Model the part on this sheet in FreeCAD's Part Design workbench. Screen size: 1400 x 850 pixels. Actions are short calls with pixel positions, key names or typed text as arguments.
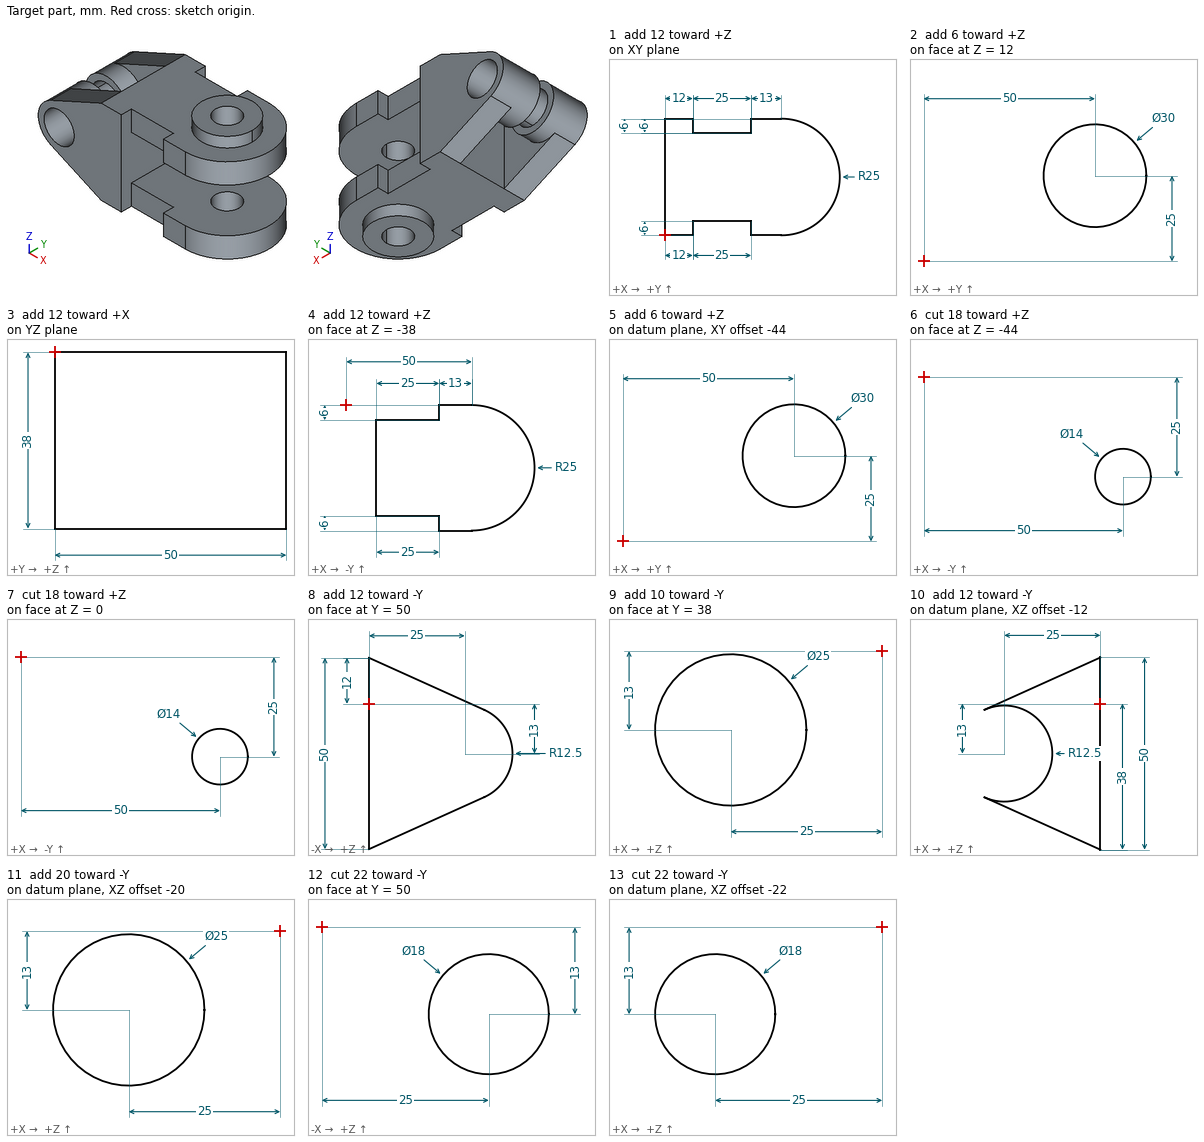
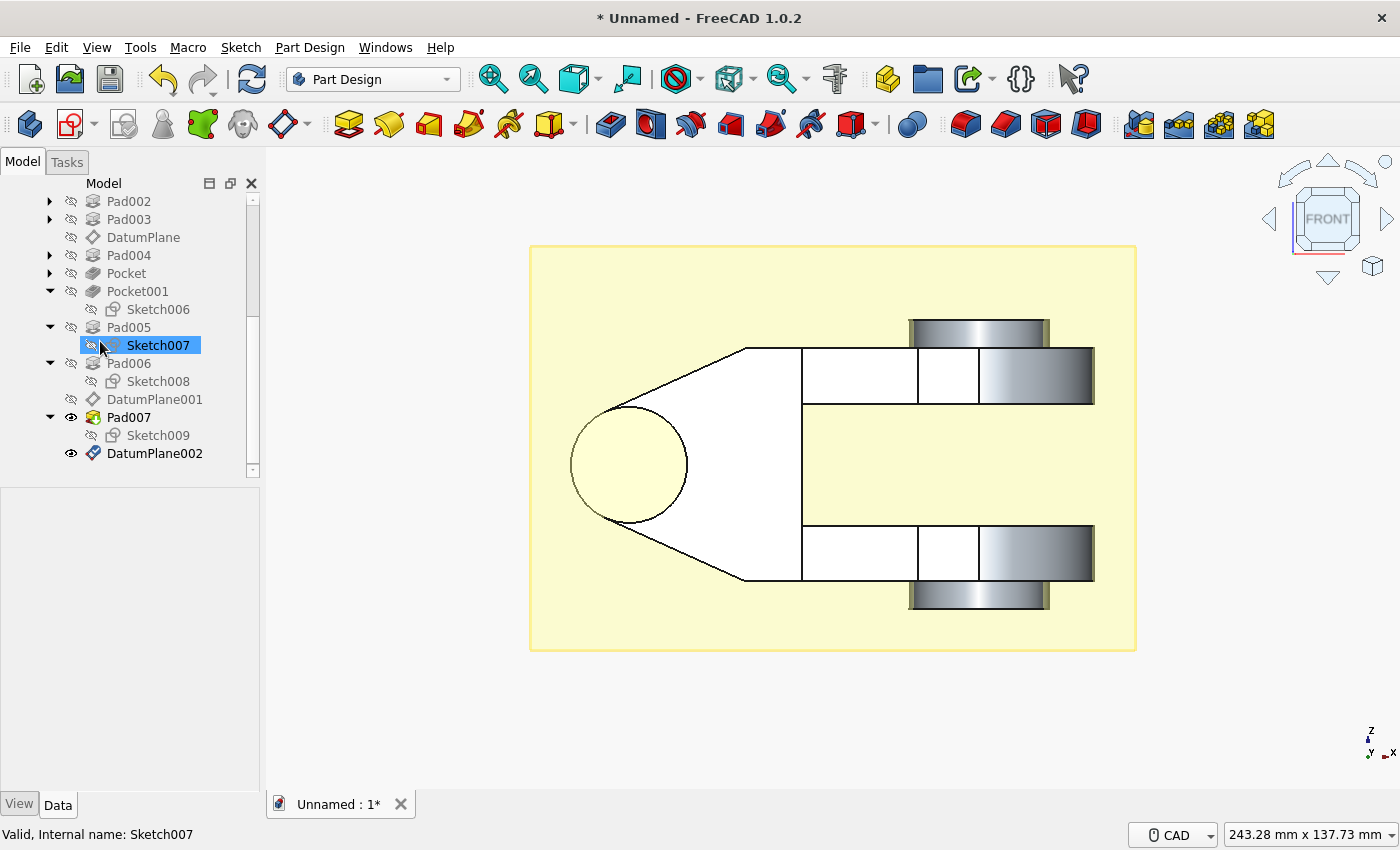
click(116, 453)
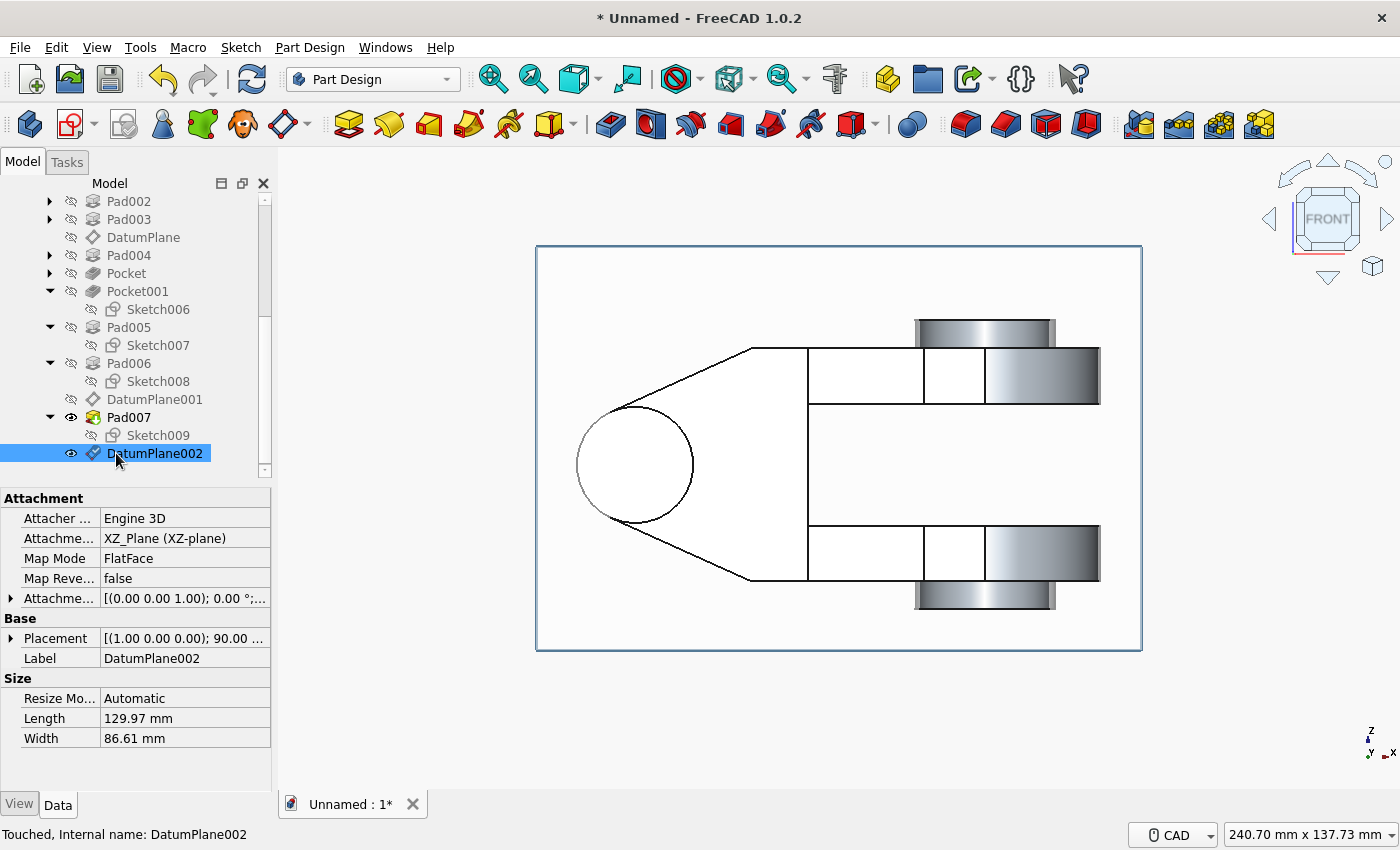
click(70, 124)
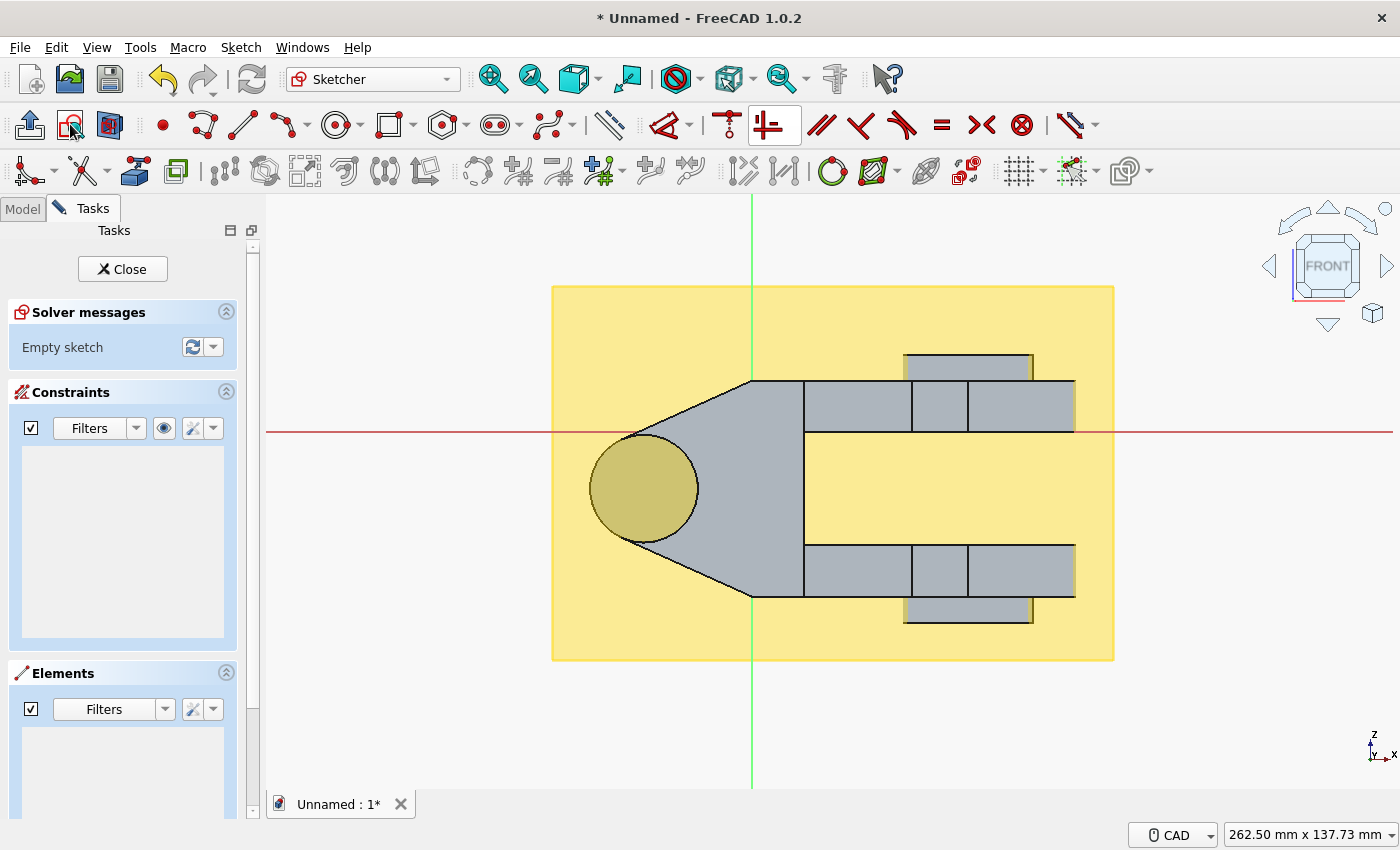
key(q)
key(s)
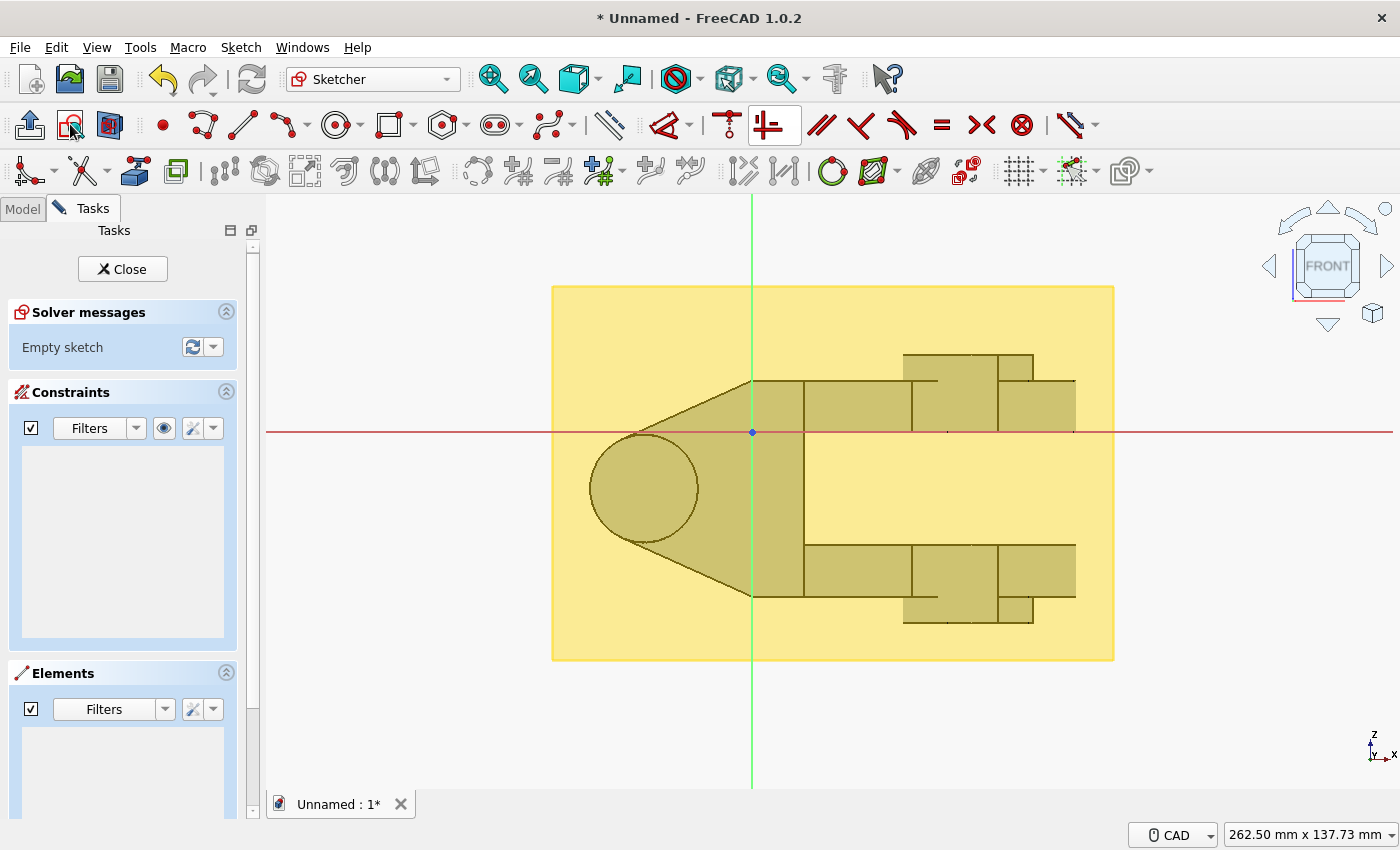
scroll(631, 486, up, 6)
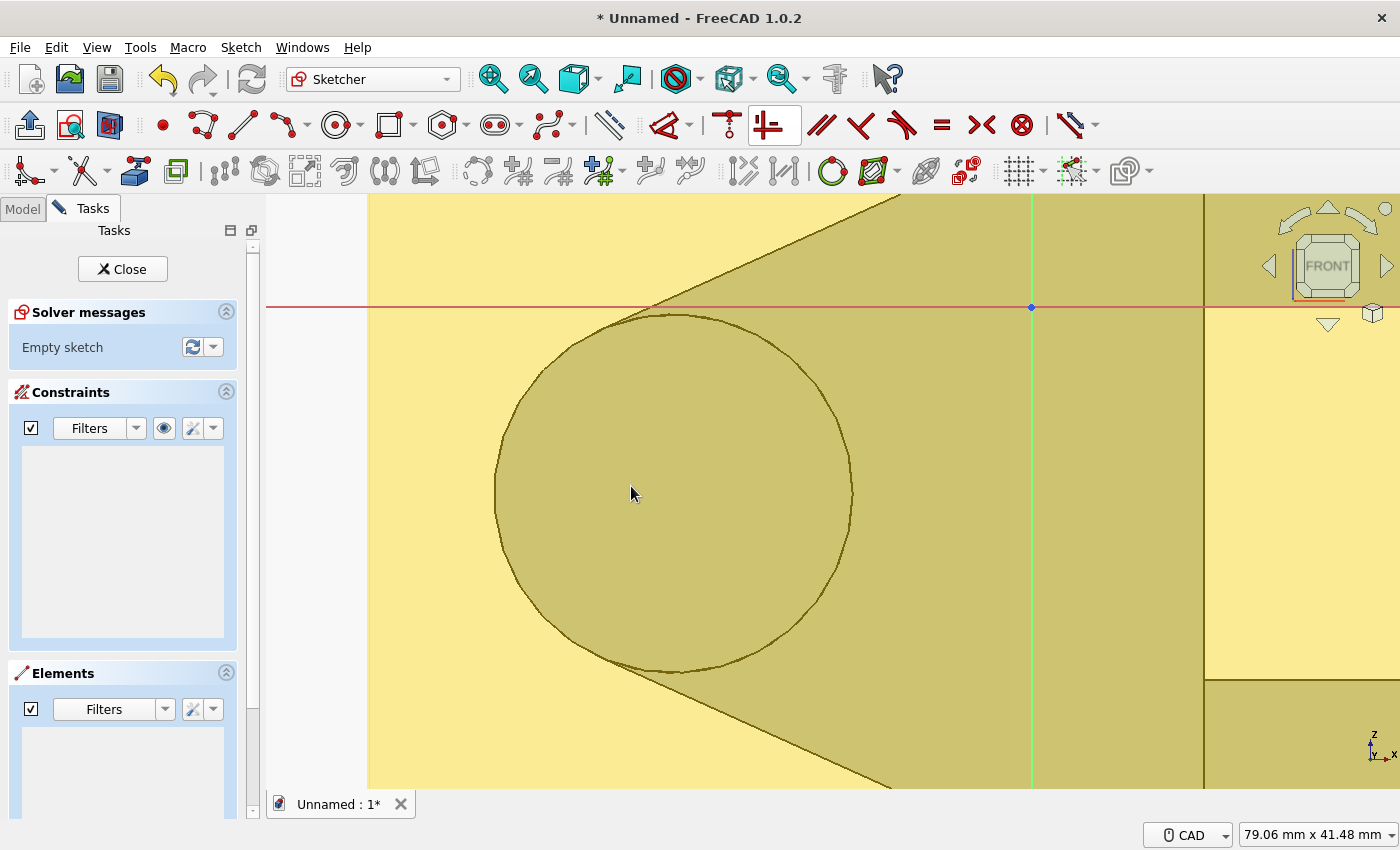
click(336, 126)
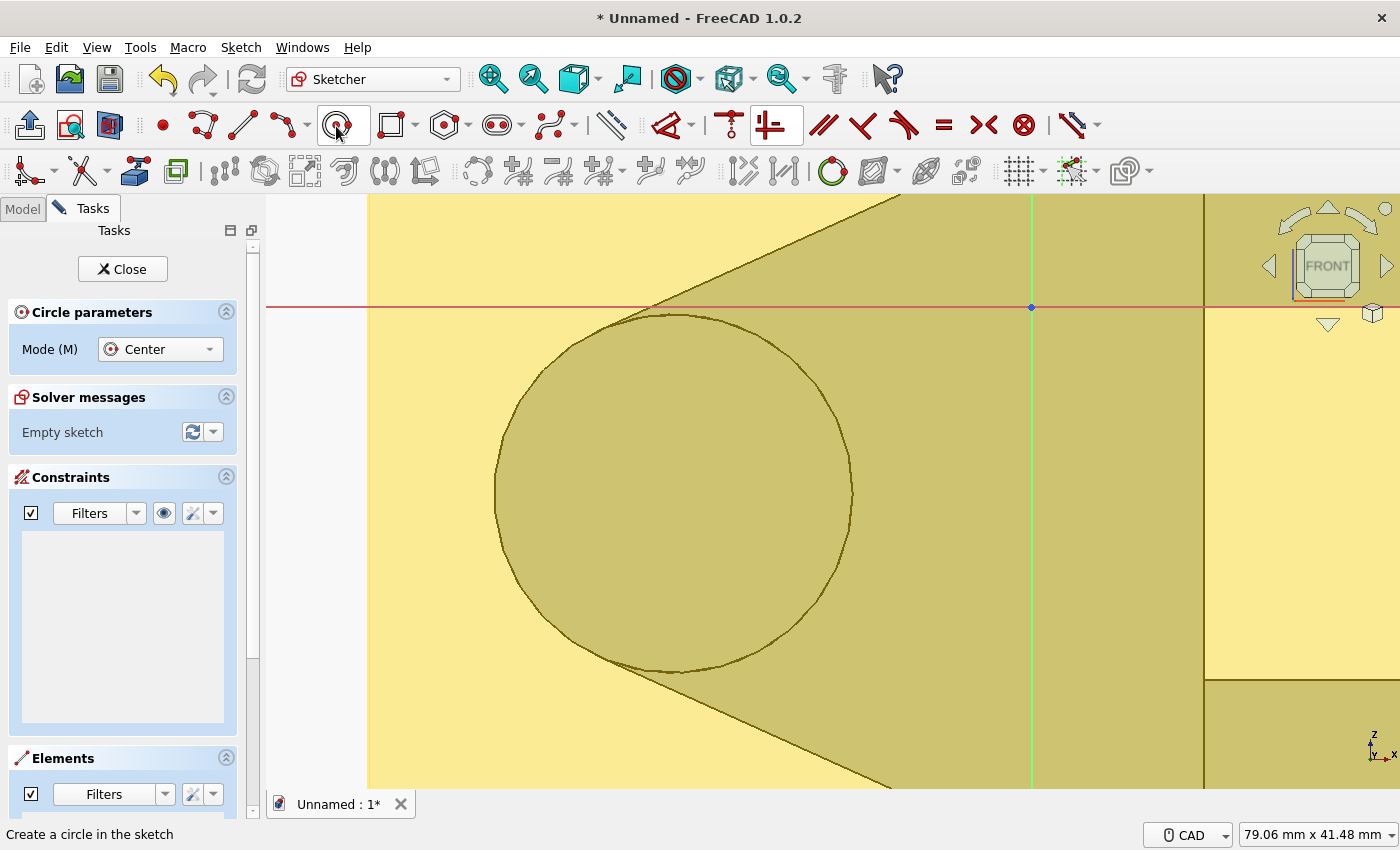
click(673, 494)
click(800, 367)
key(Escape)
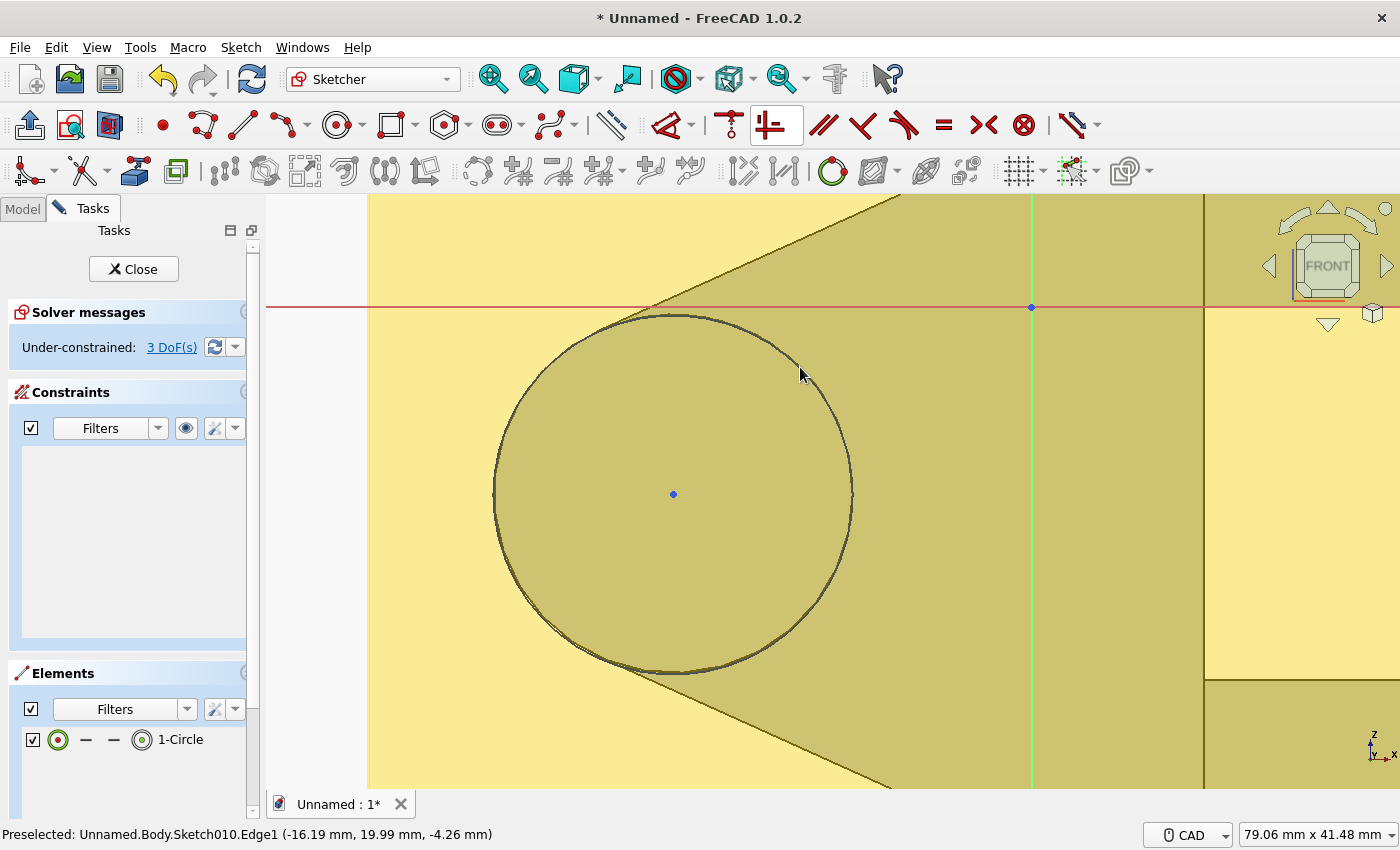
click(666, 126)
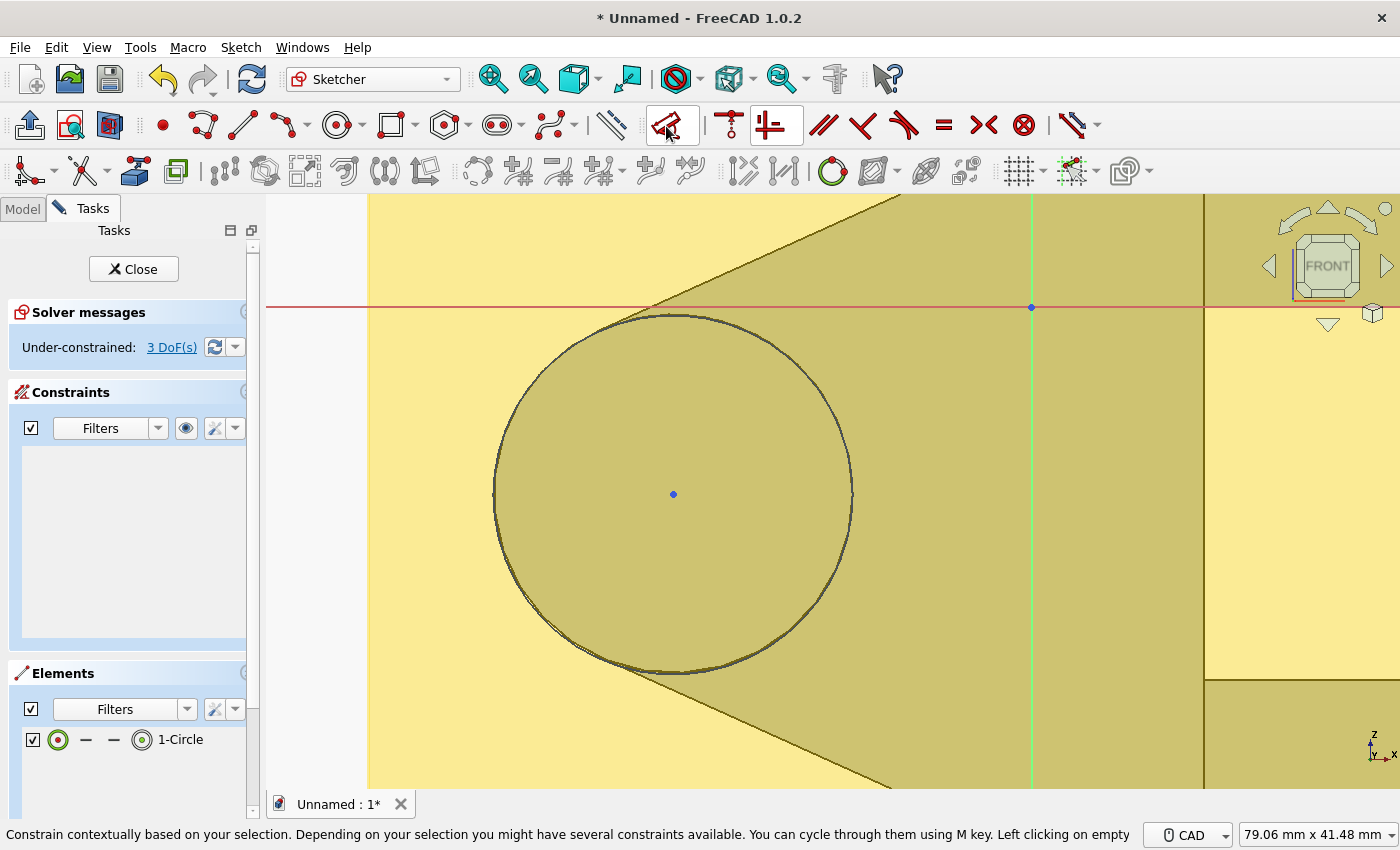
click(800, 368)
click(823, 345)